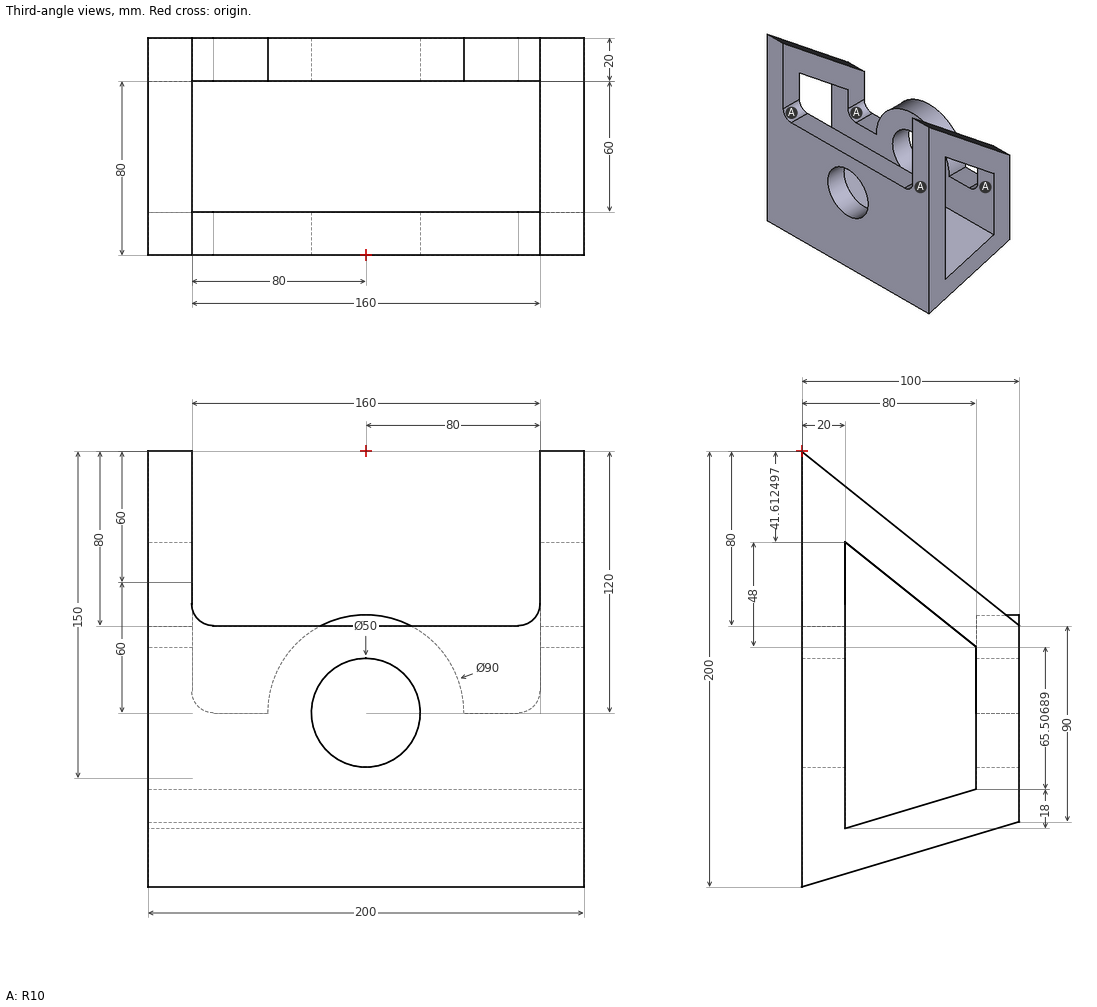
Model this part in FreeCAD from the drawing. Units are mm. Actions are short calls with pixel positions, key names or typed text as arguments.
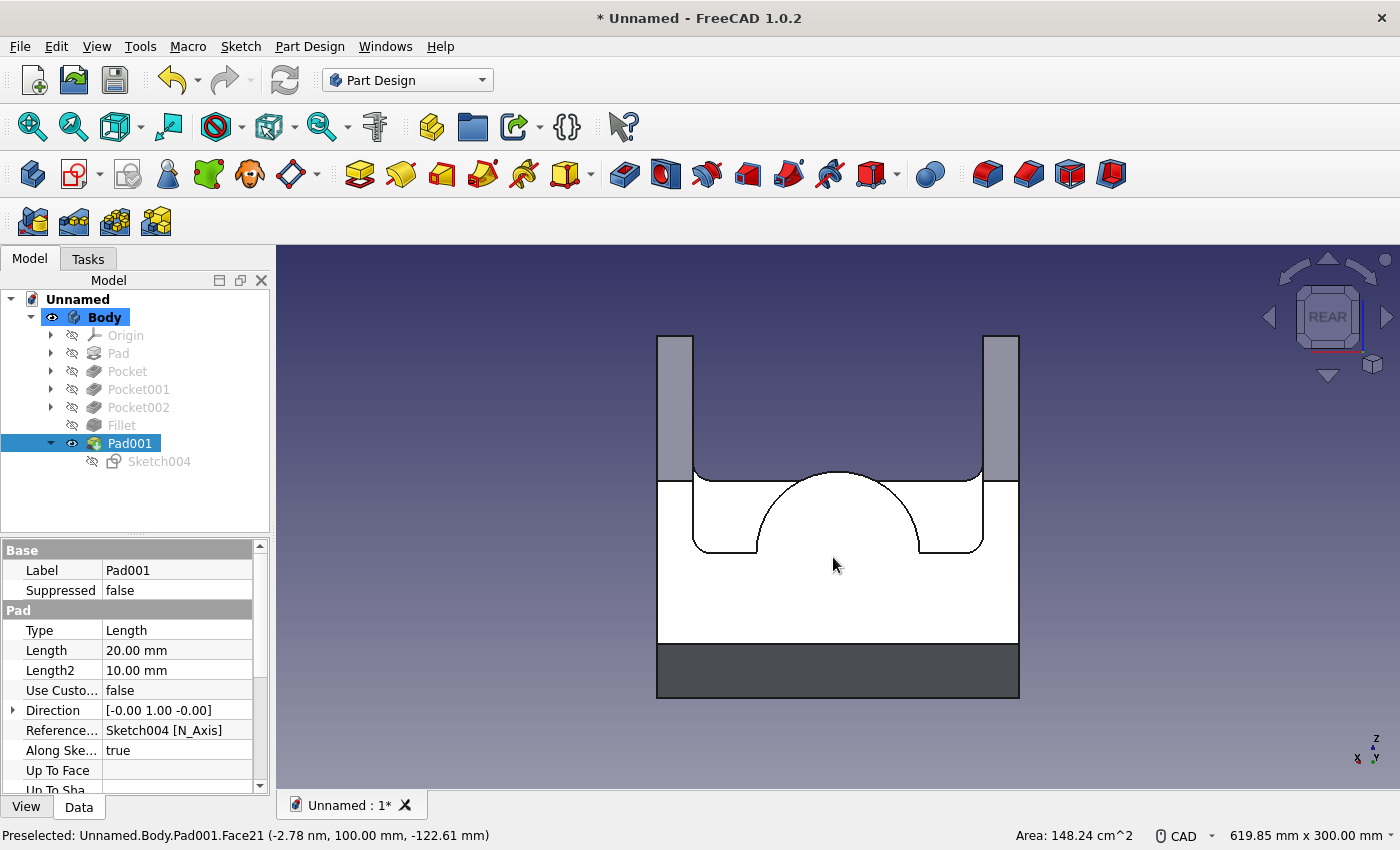
click(74, 174)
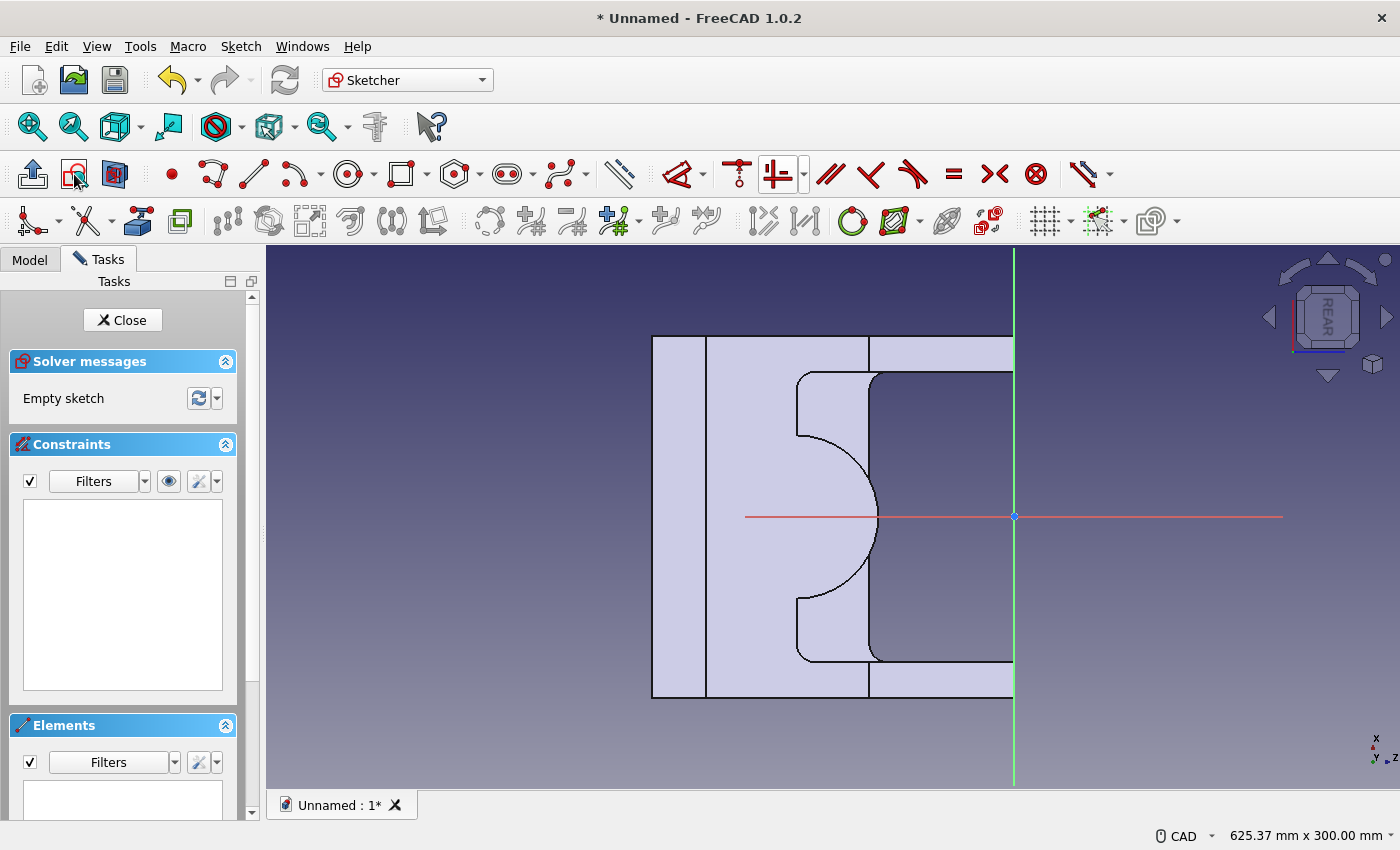
scroll(807, 517, up, 7)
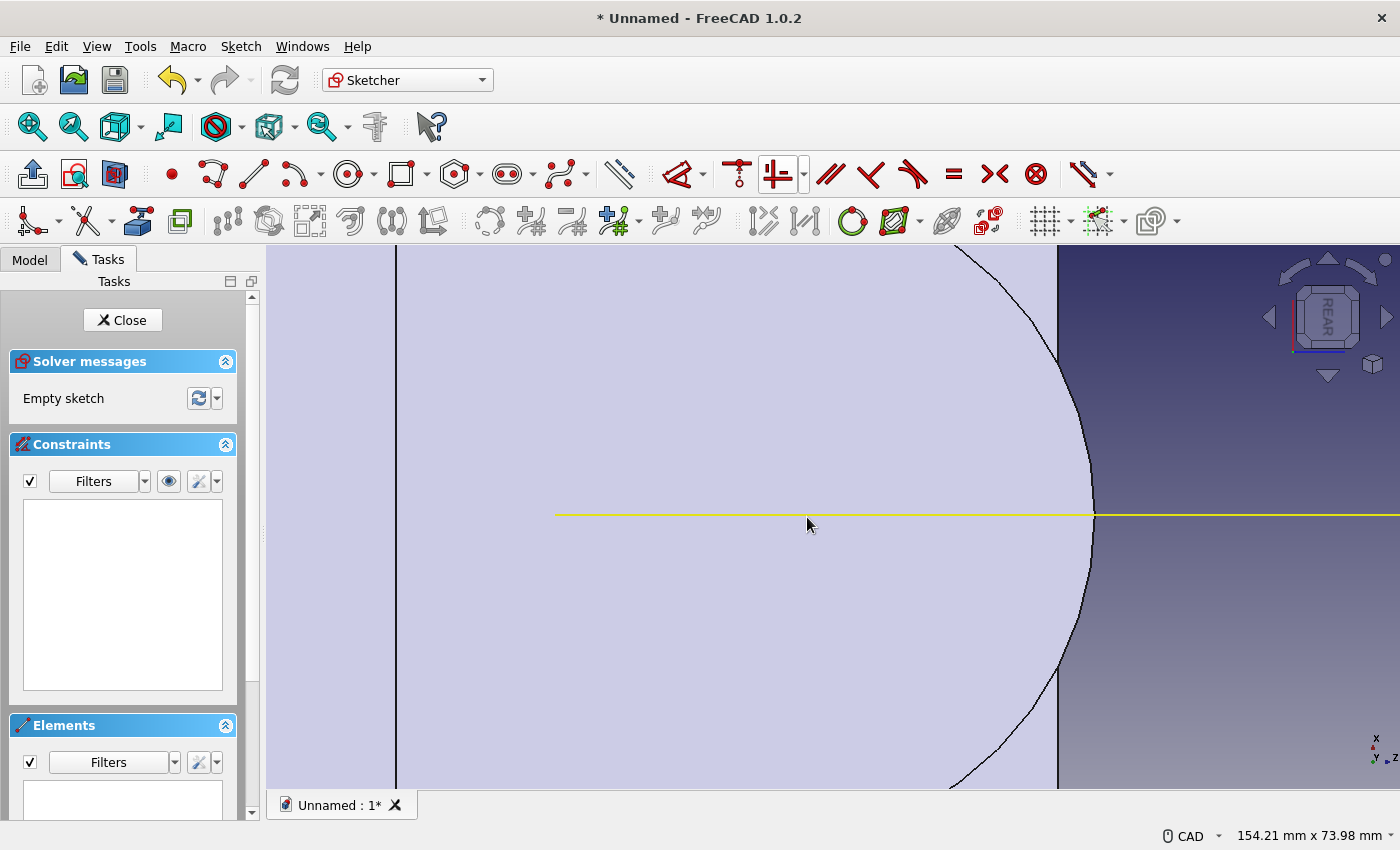
click(348, 174)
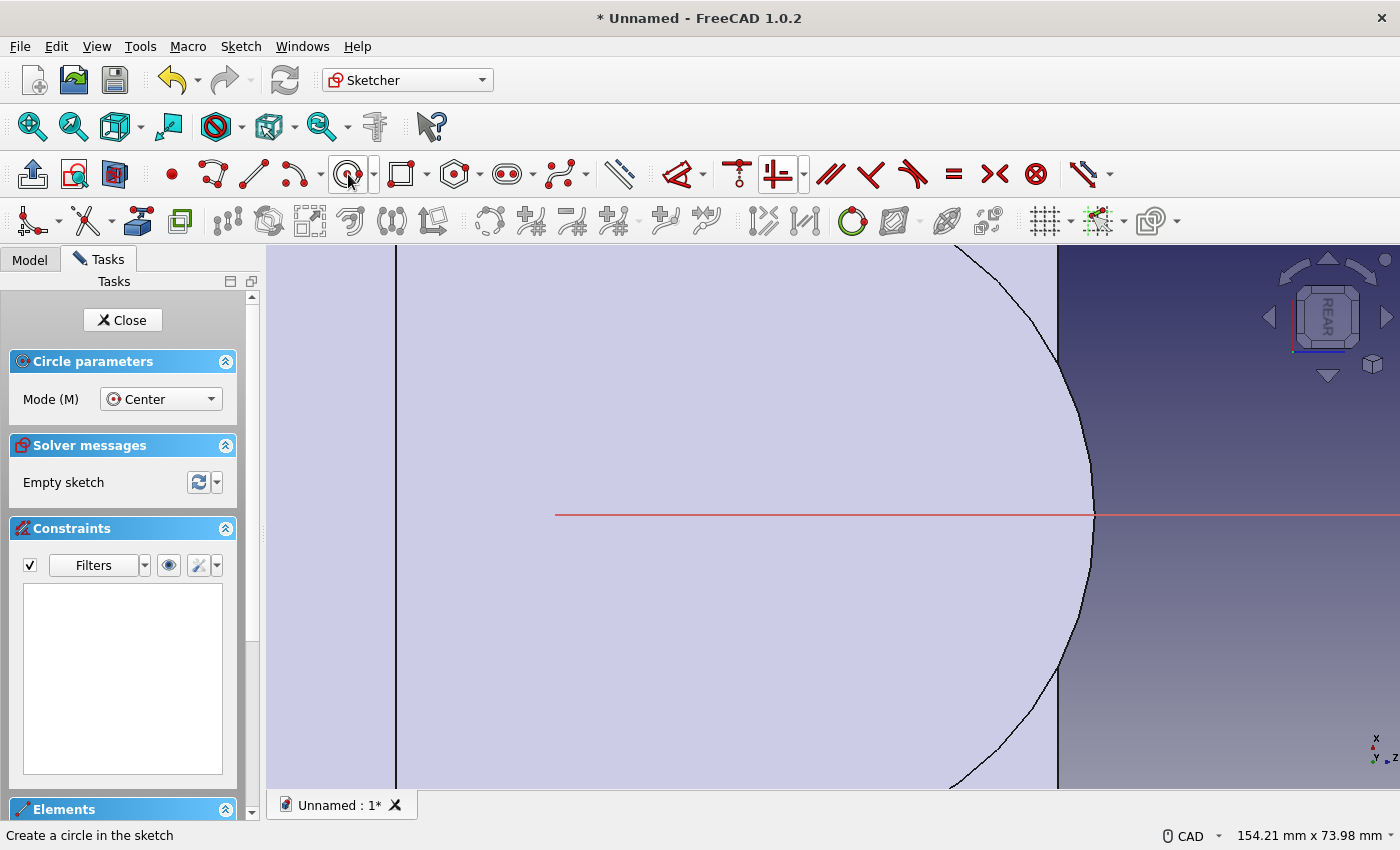
click(764, 515)
move(894, 385)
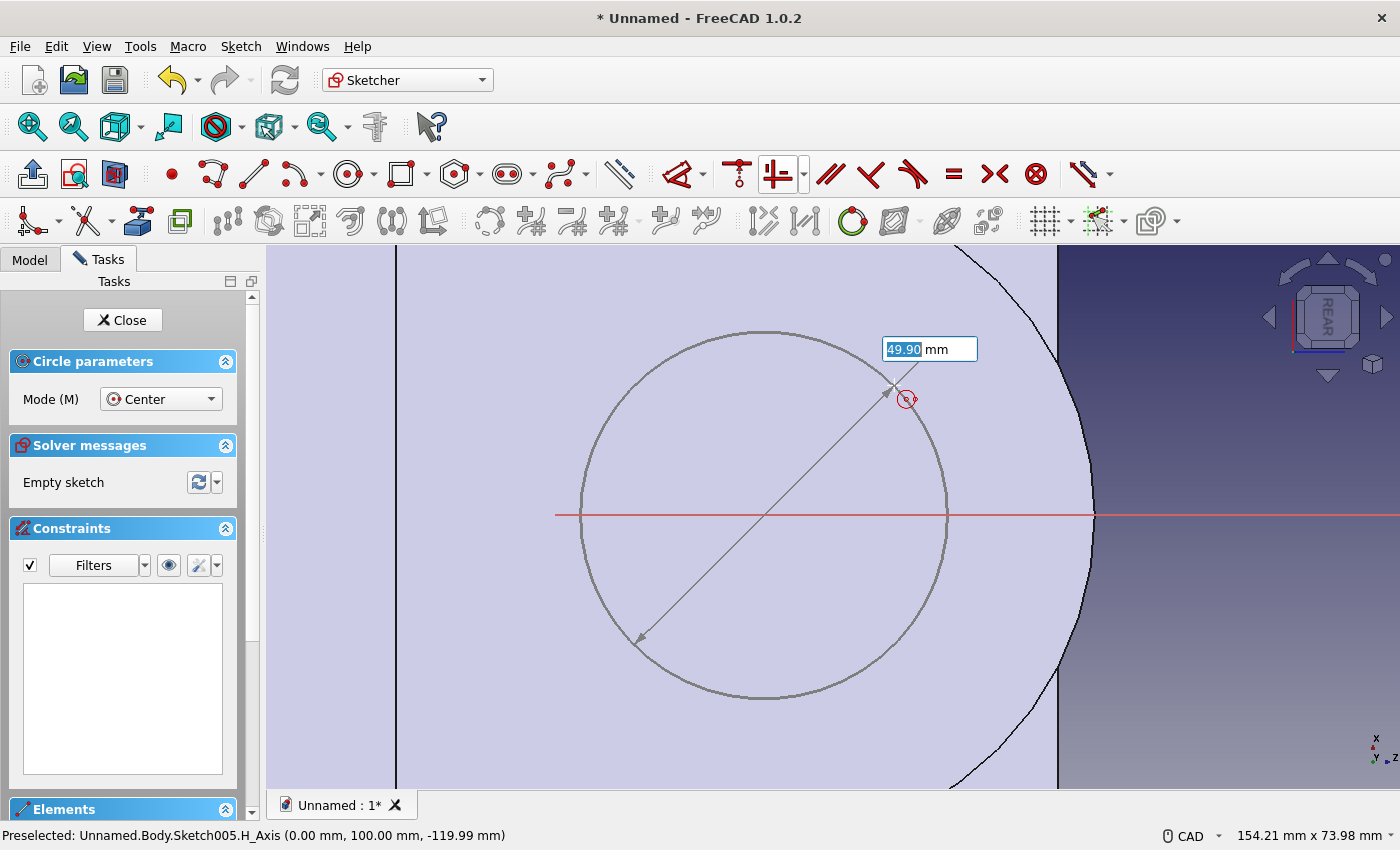
text(50)
key(Return)
key(Escape)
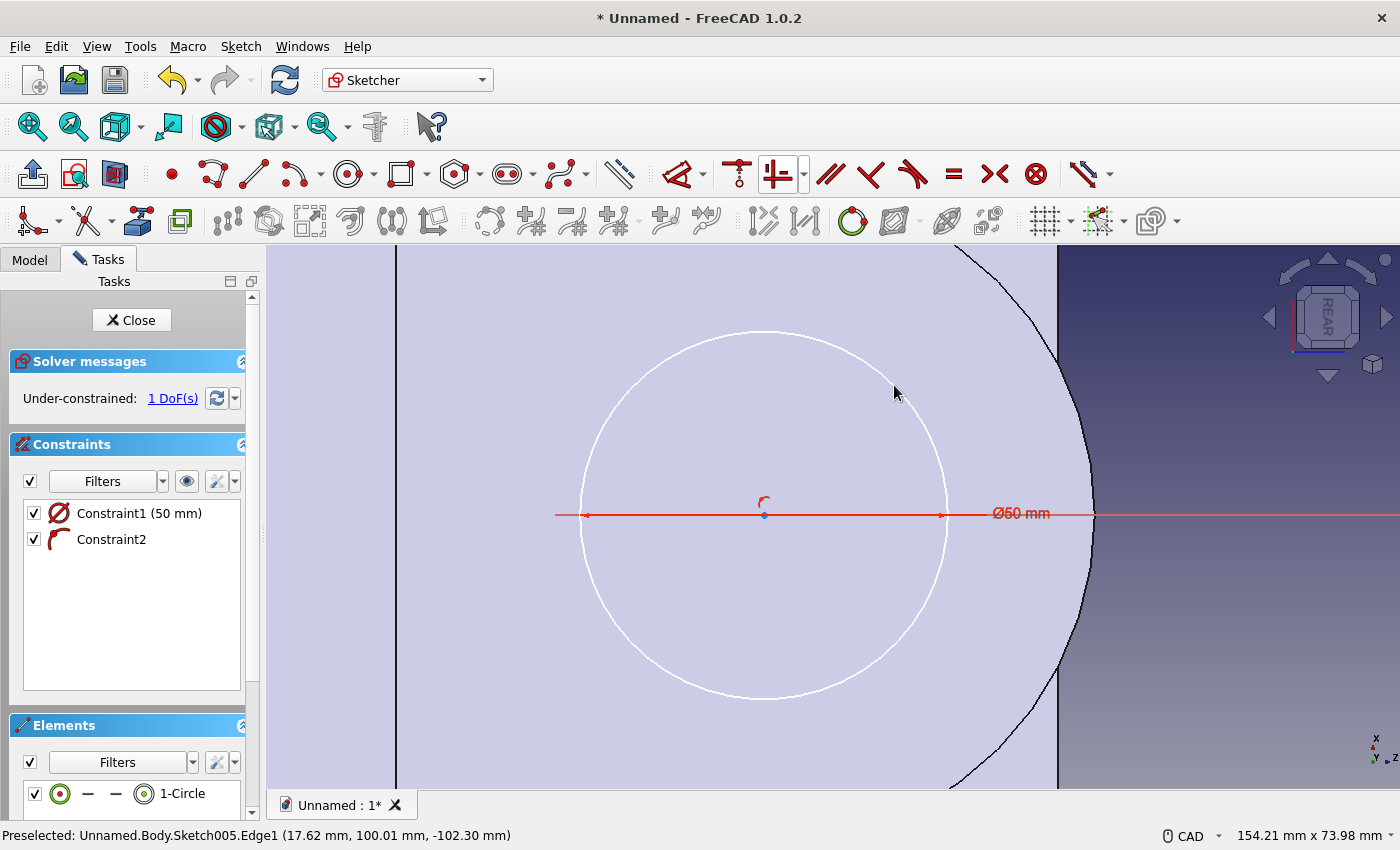
key(d)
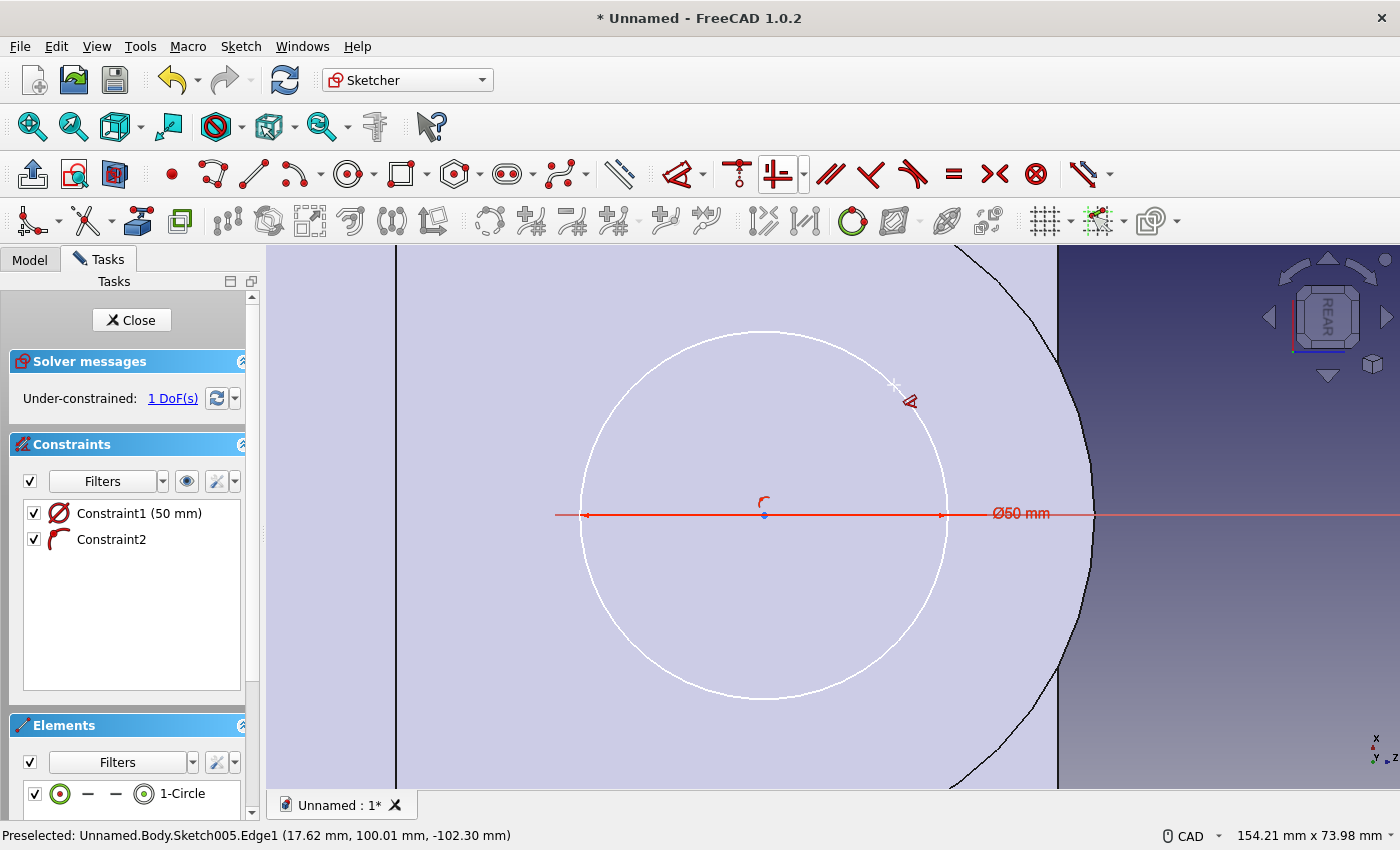
click(764, 515)
click(1000, 549)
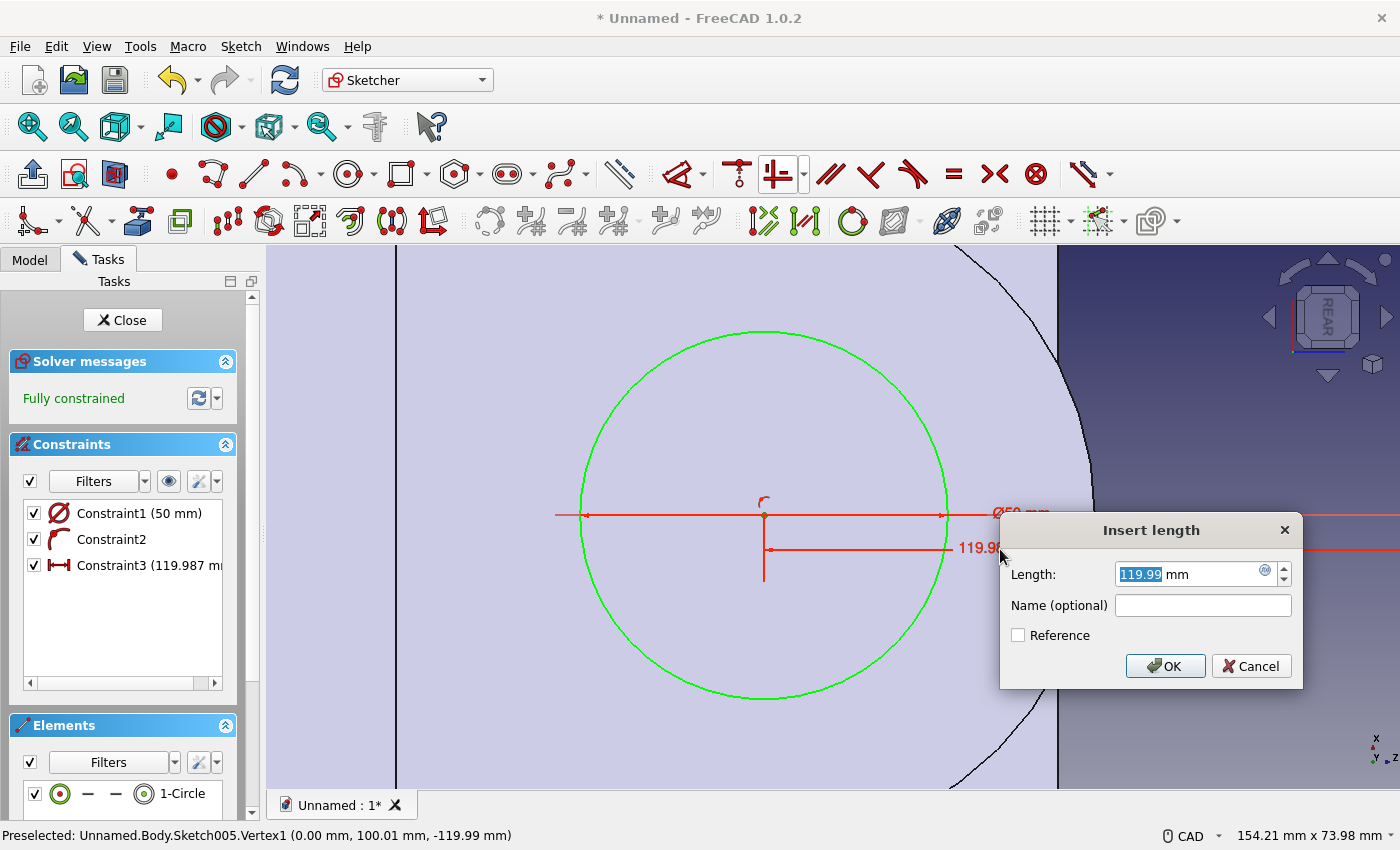
text(120)
key(Return)
key(Escape)